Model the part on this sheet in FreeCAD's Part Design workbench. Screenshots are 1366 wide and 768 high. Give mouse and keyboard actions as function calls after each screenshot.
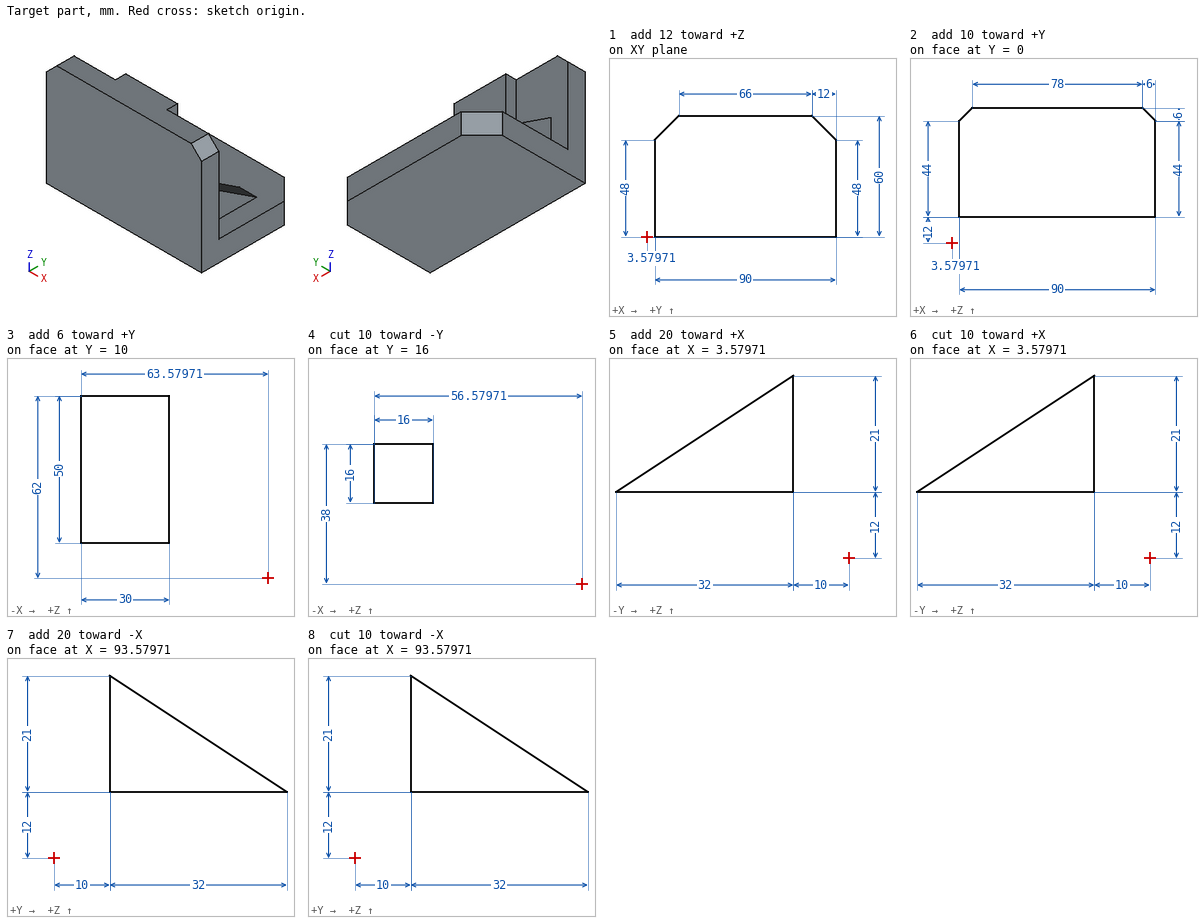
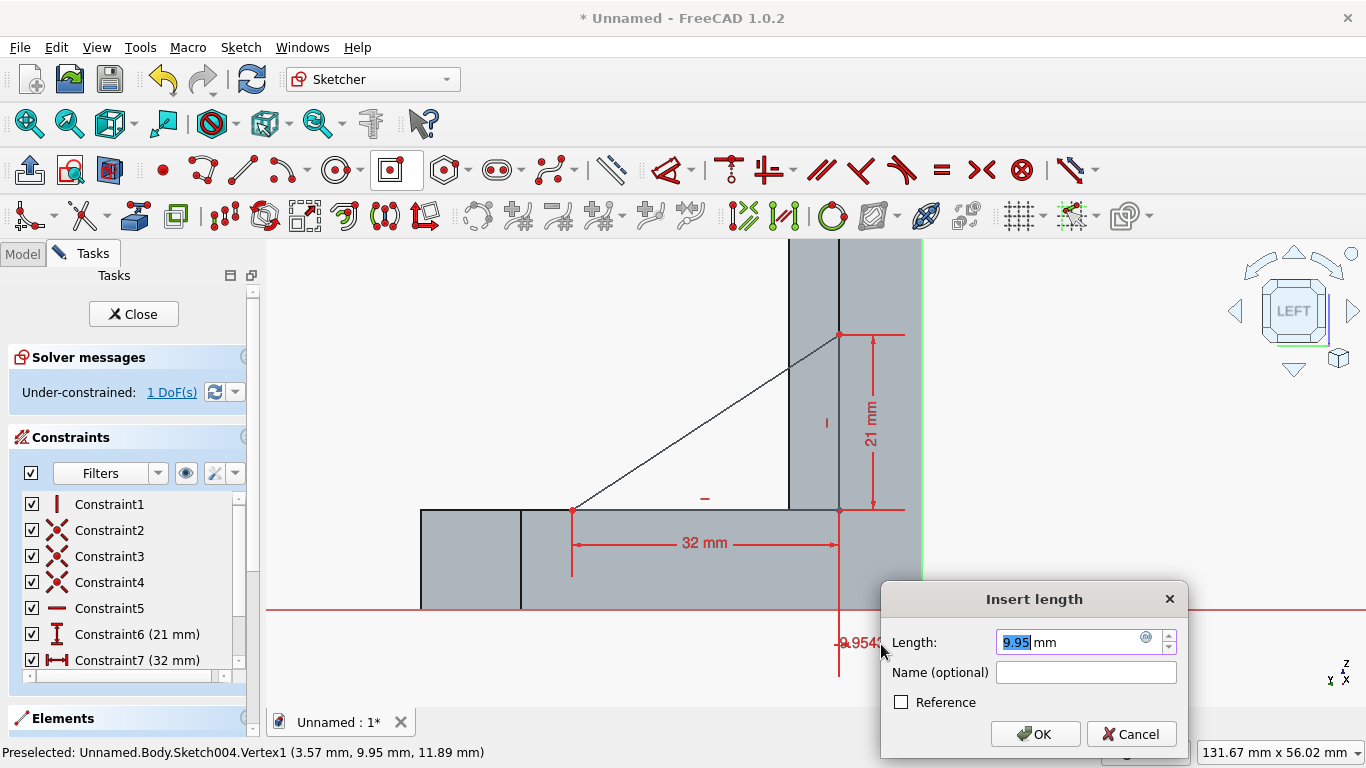
text(10)
key(Return)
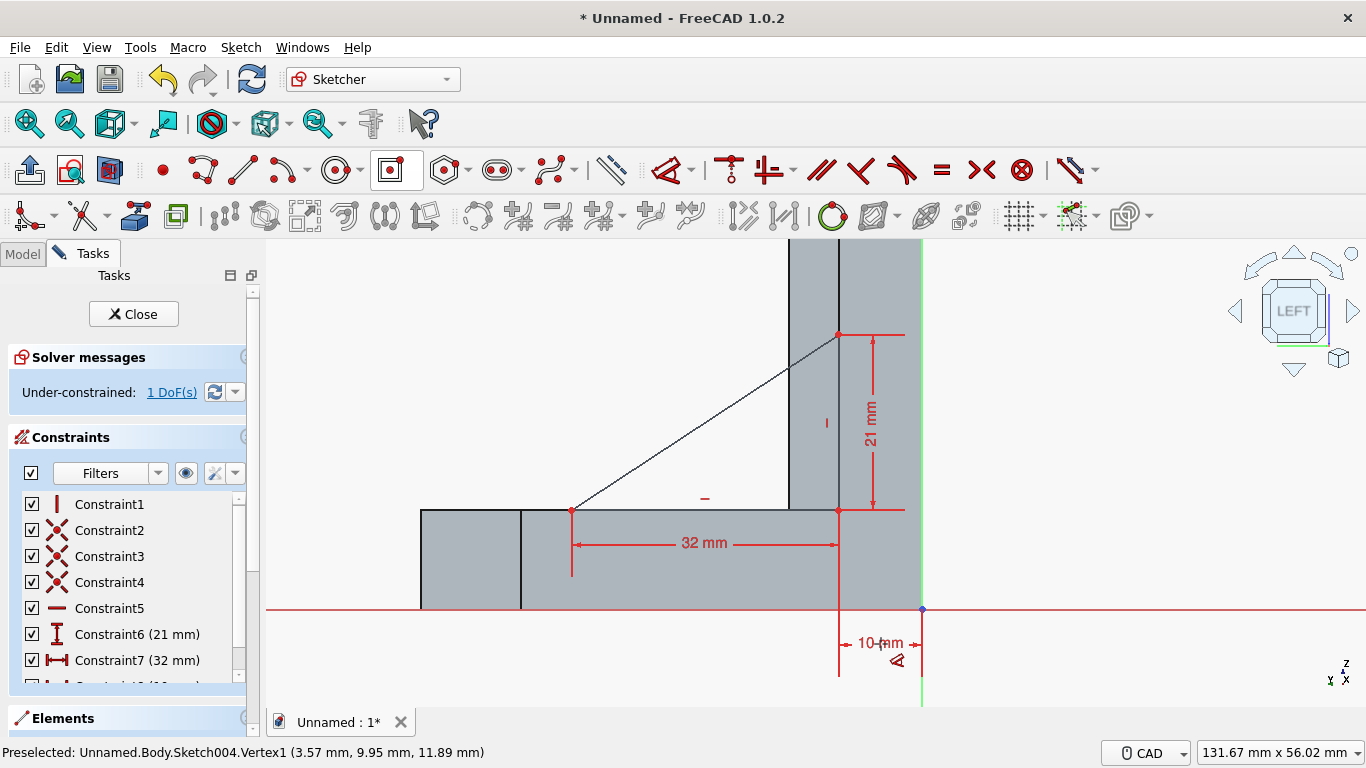
click(839, 510)
click(956, 560)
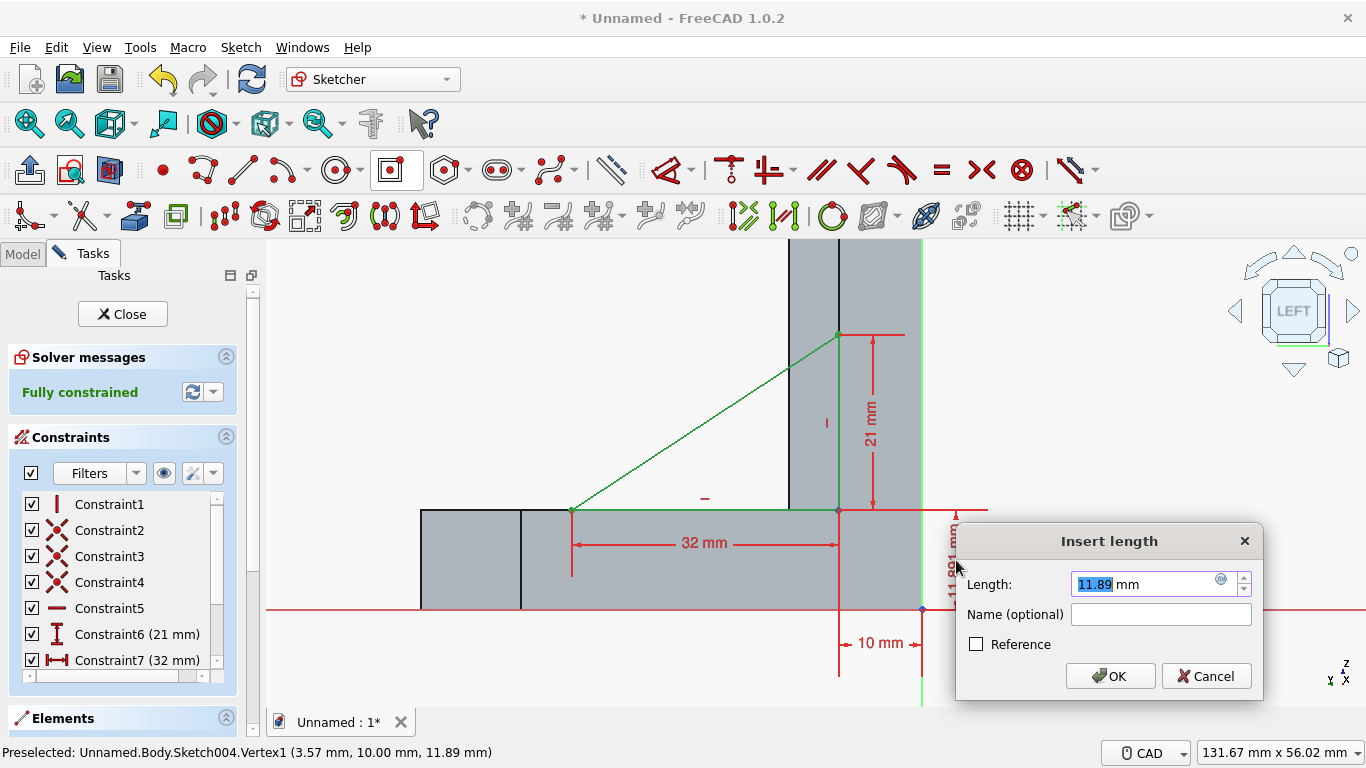
text(12)
key(Return)
key(Escape)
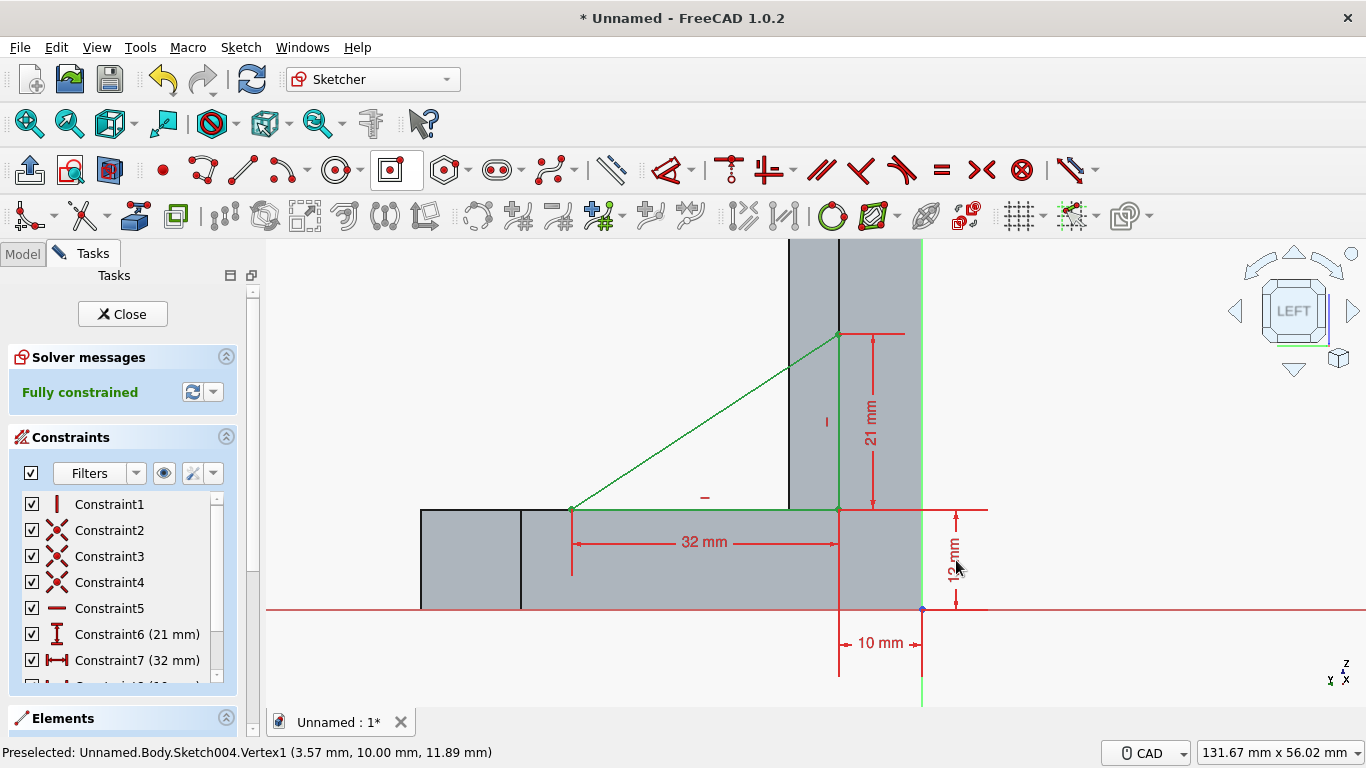
click(123, 314)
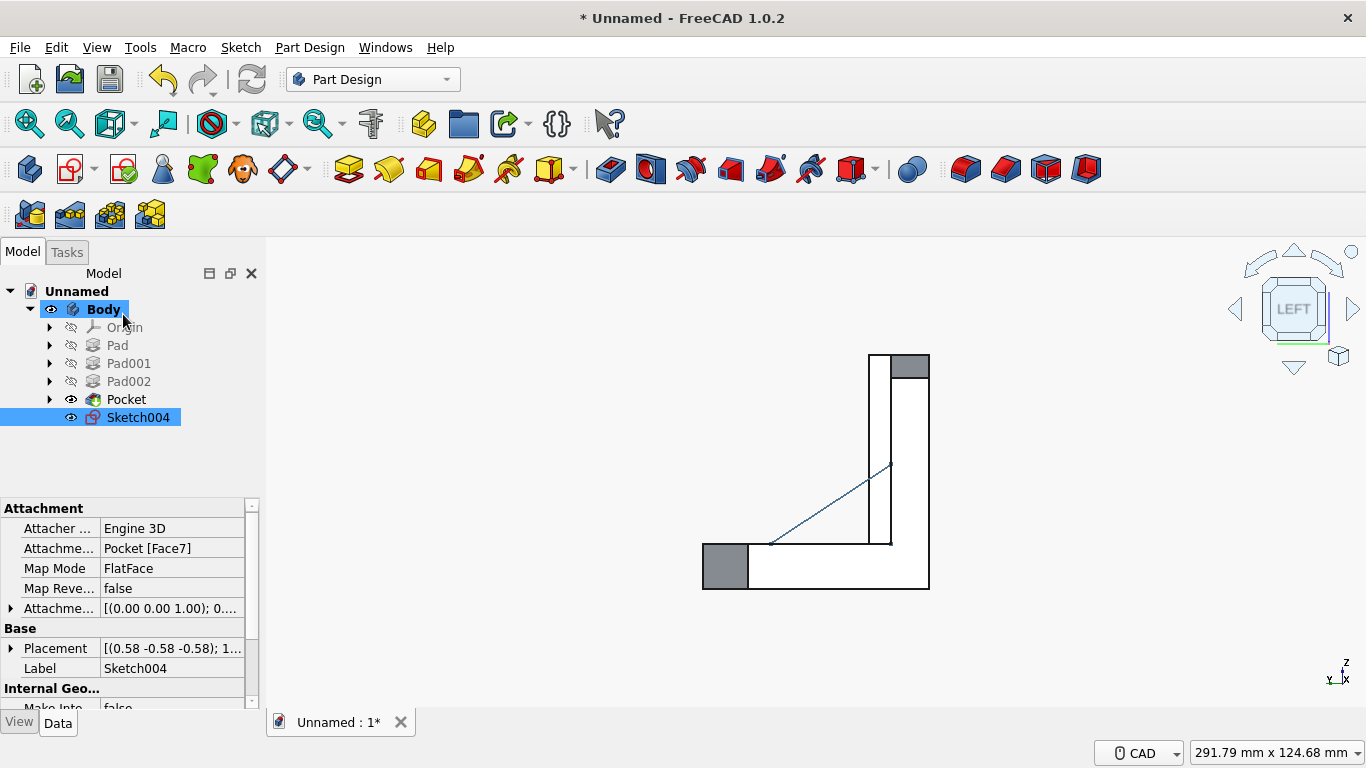
click(350, 170)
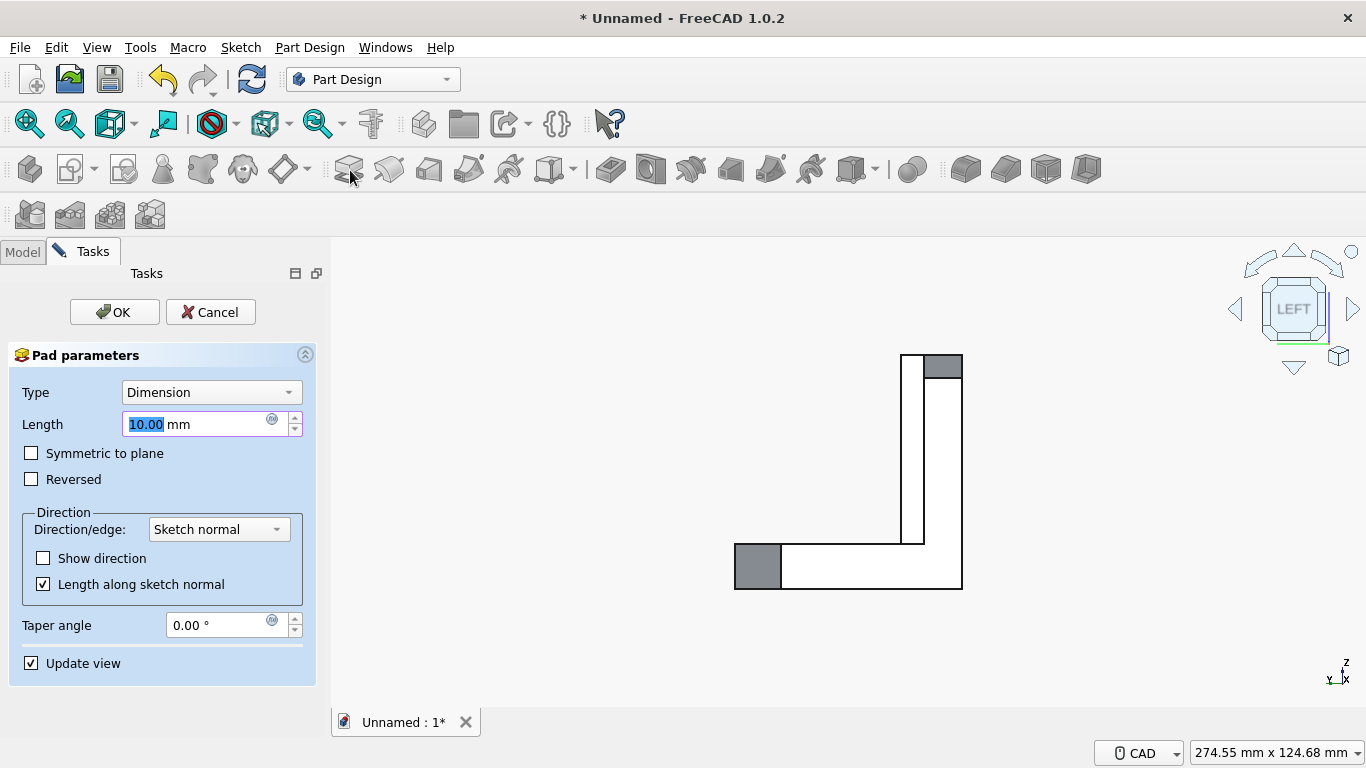
text(20)
key(Tab)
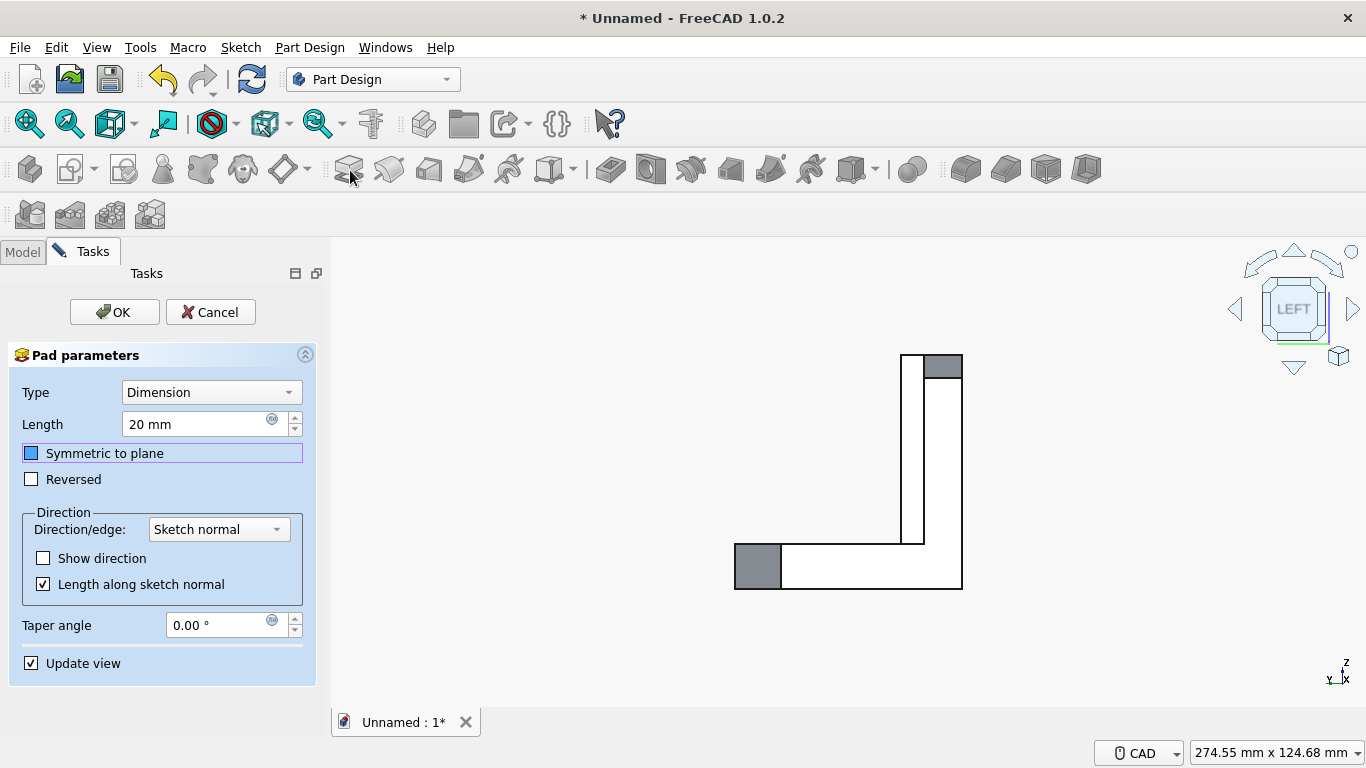
click(30, 479)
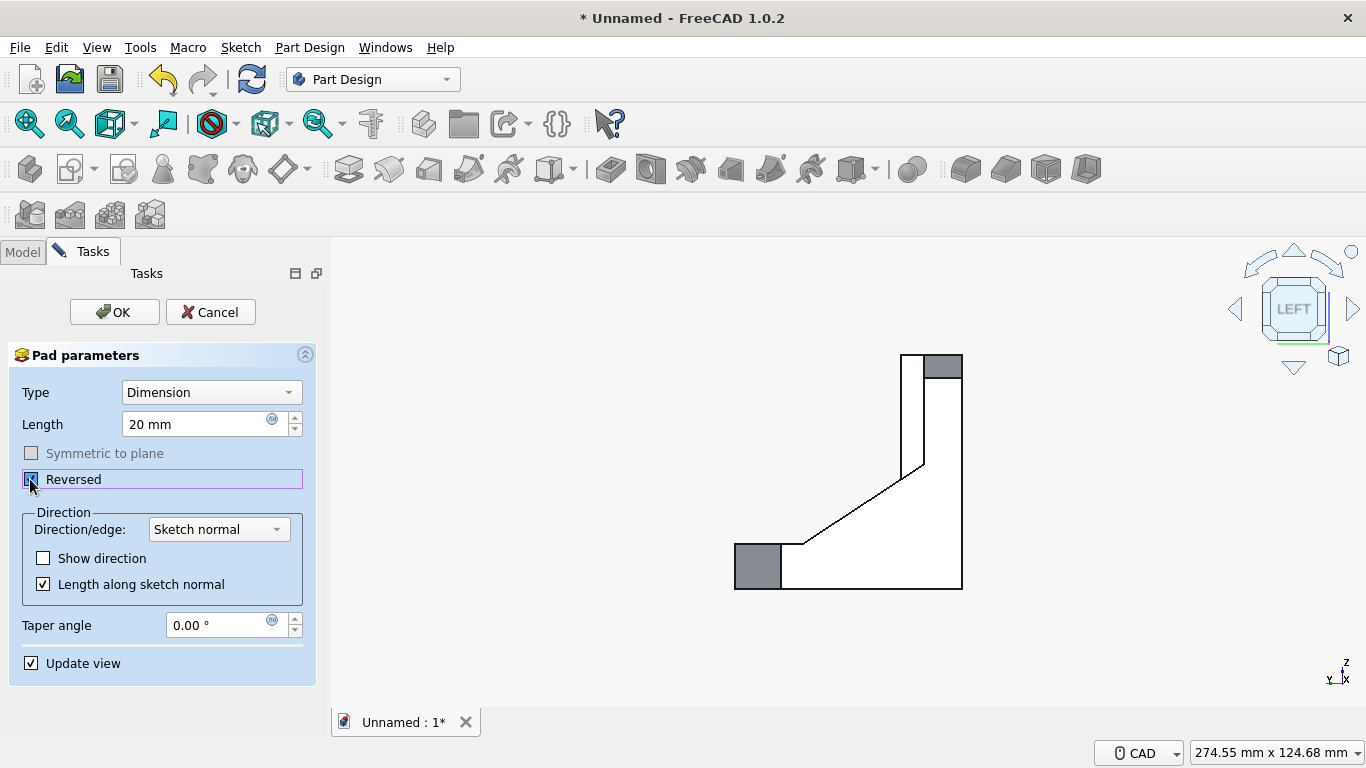
click(115, 312)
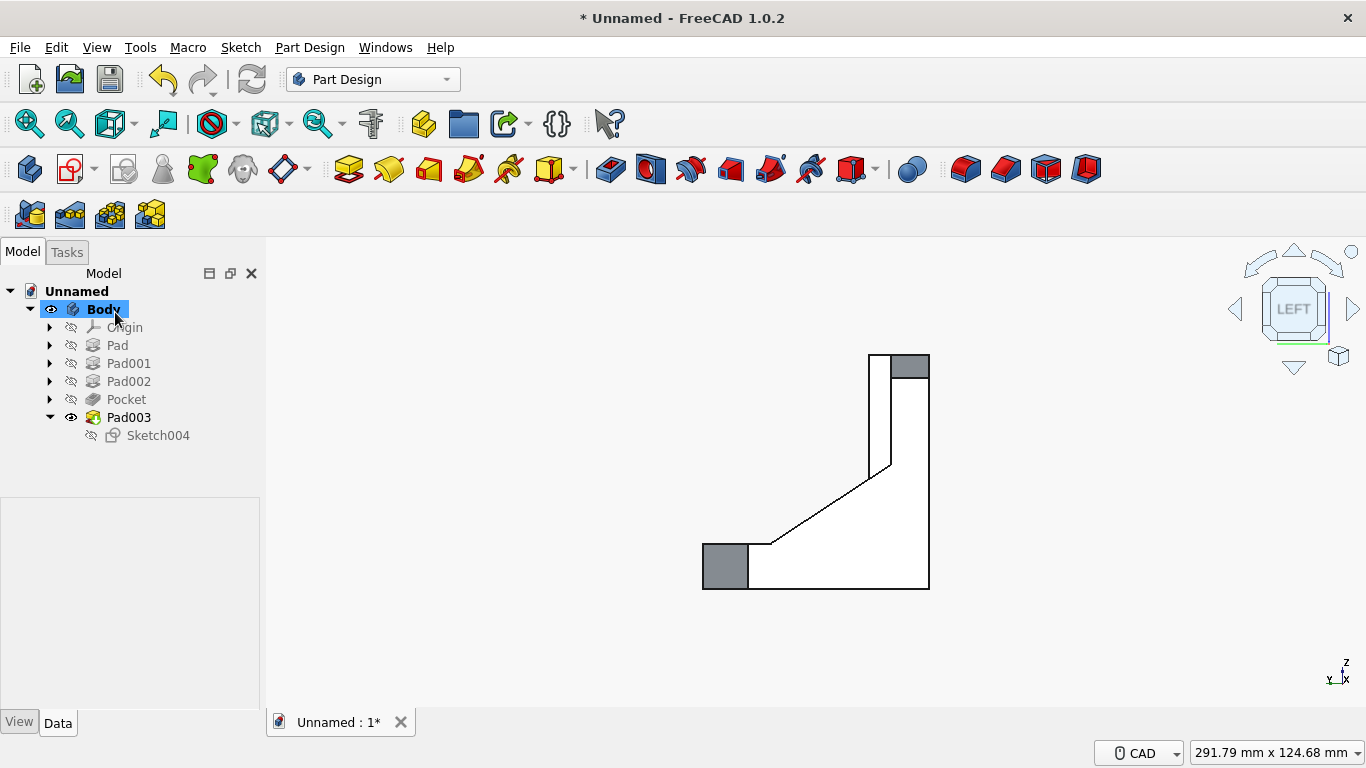
click(864, 543)